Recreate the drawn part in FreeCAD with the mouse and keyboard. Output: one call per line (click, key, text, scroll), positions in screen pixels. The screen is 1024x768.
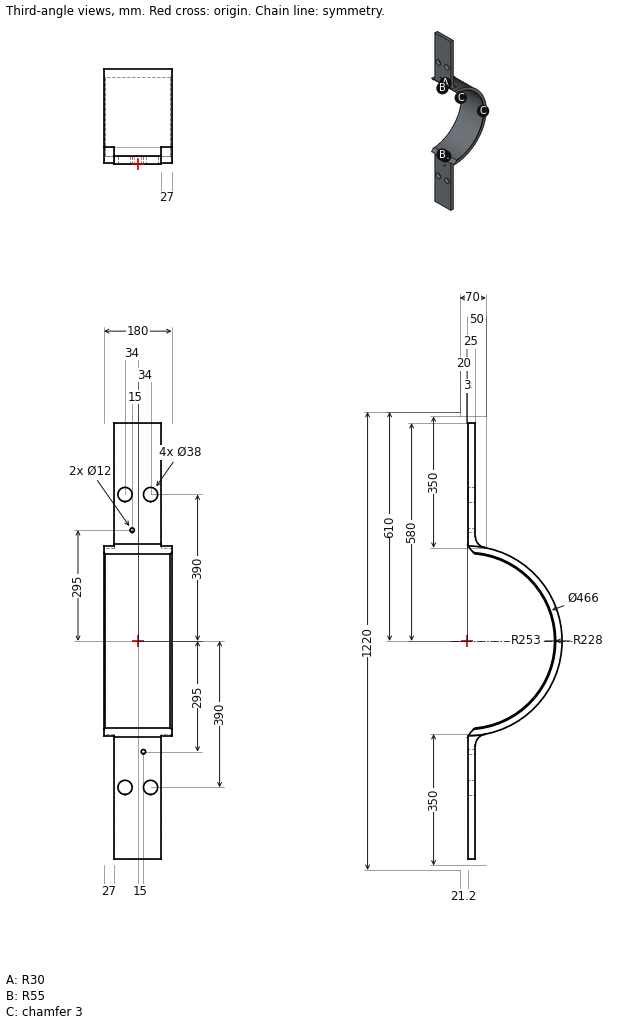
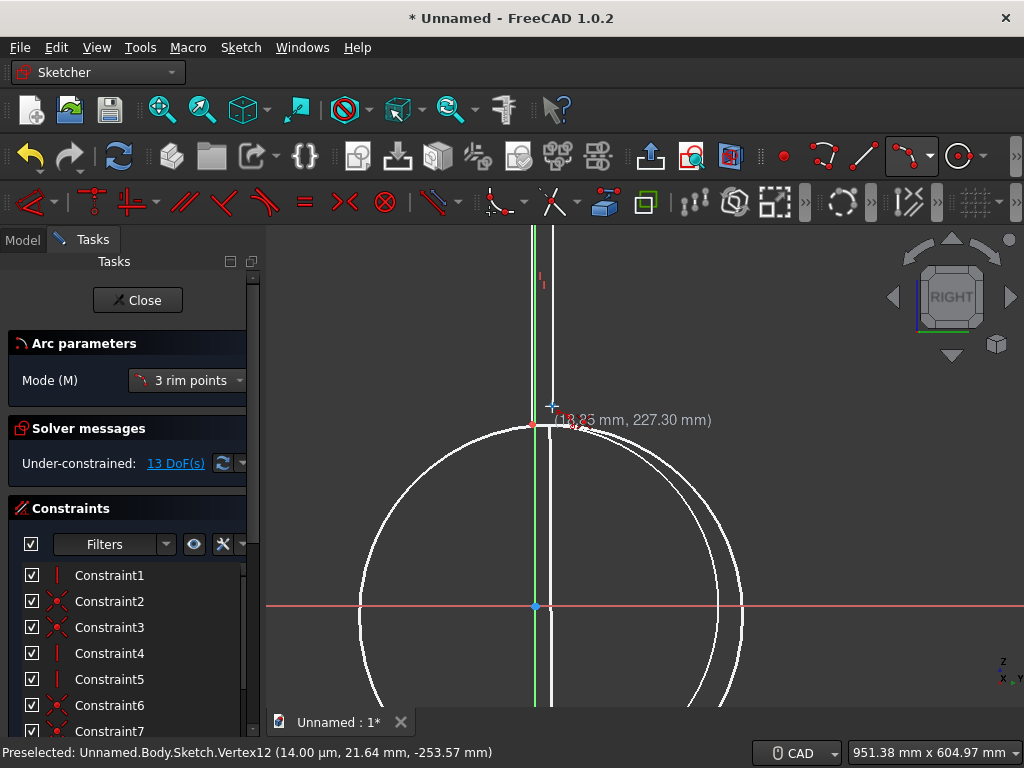
click(553, 406)
click(728, 665)
key(Escape)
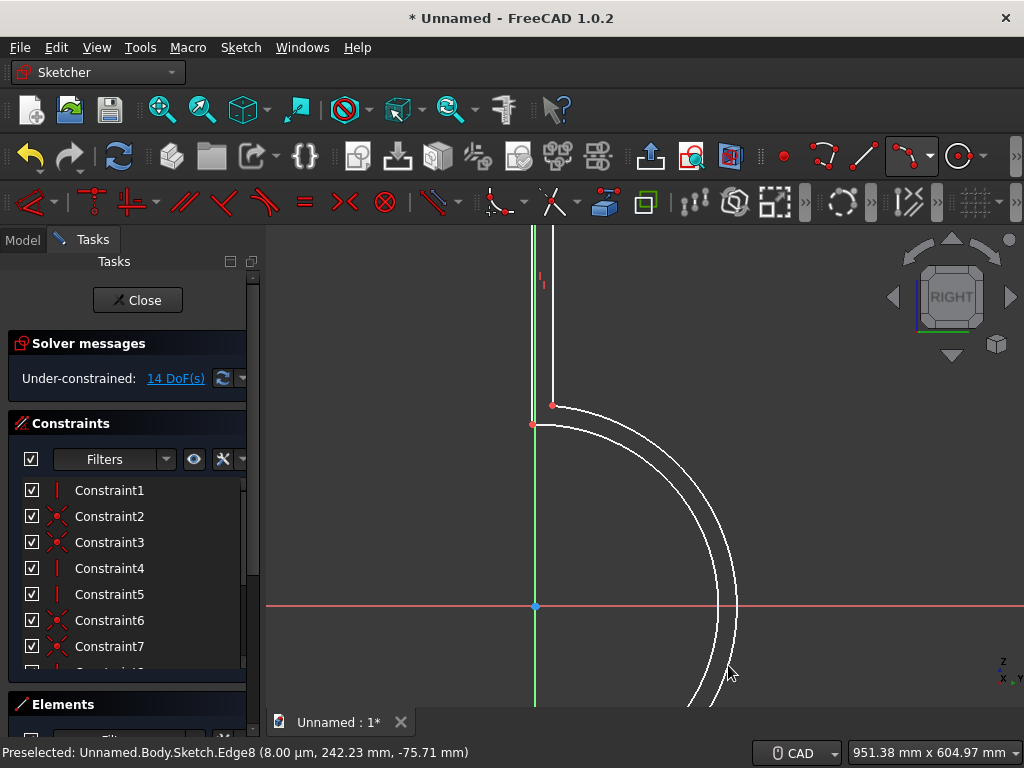
scroll(552, 406, down, 6)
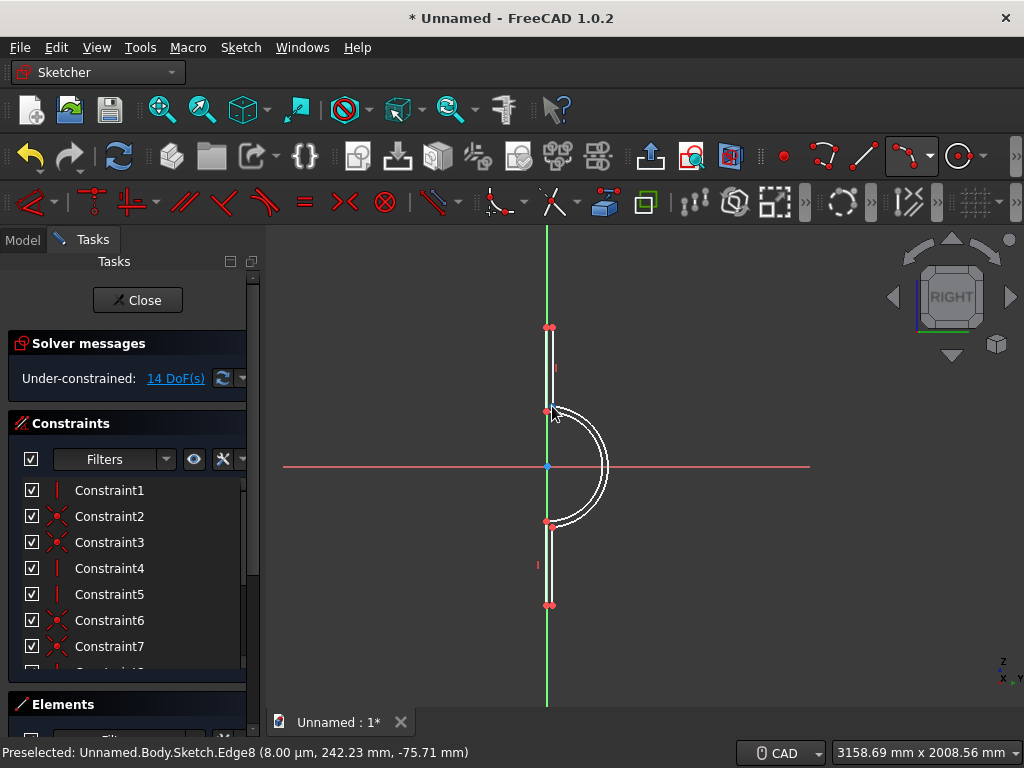
scroll(550, 328, up, 9)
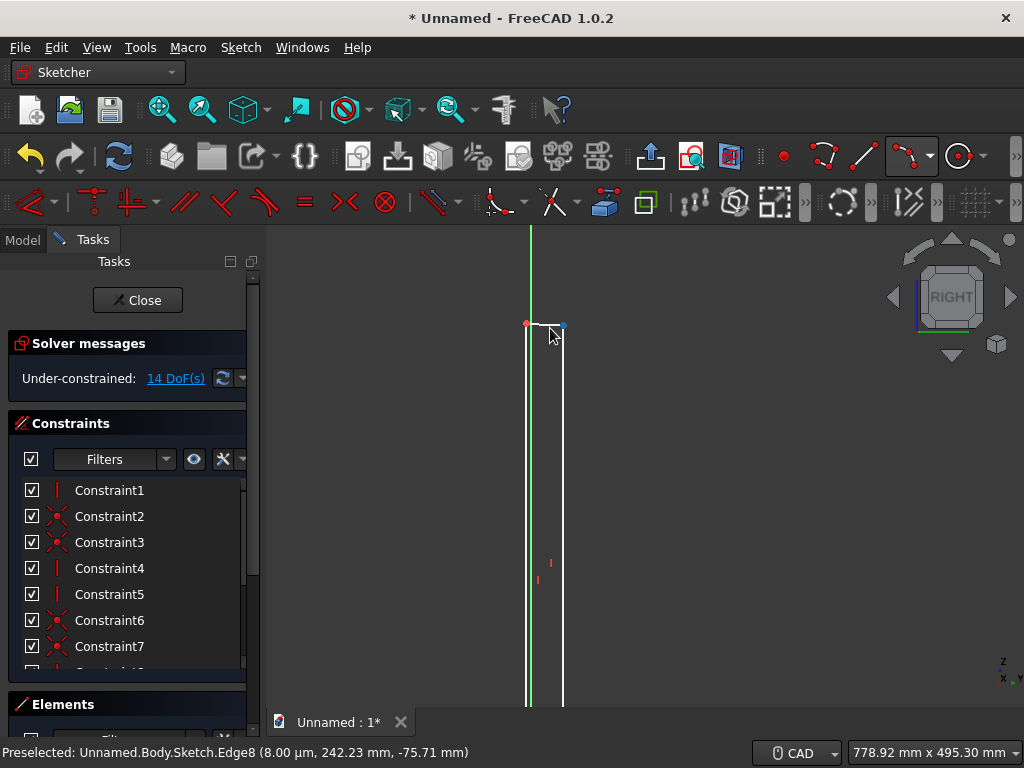
click(549, 325)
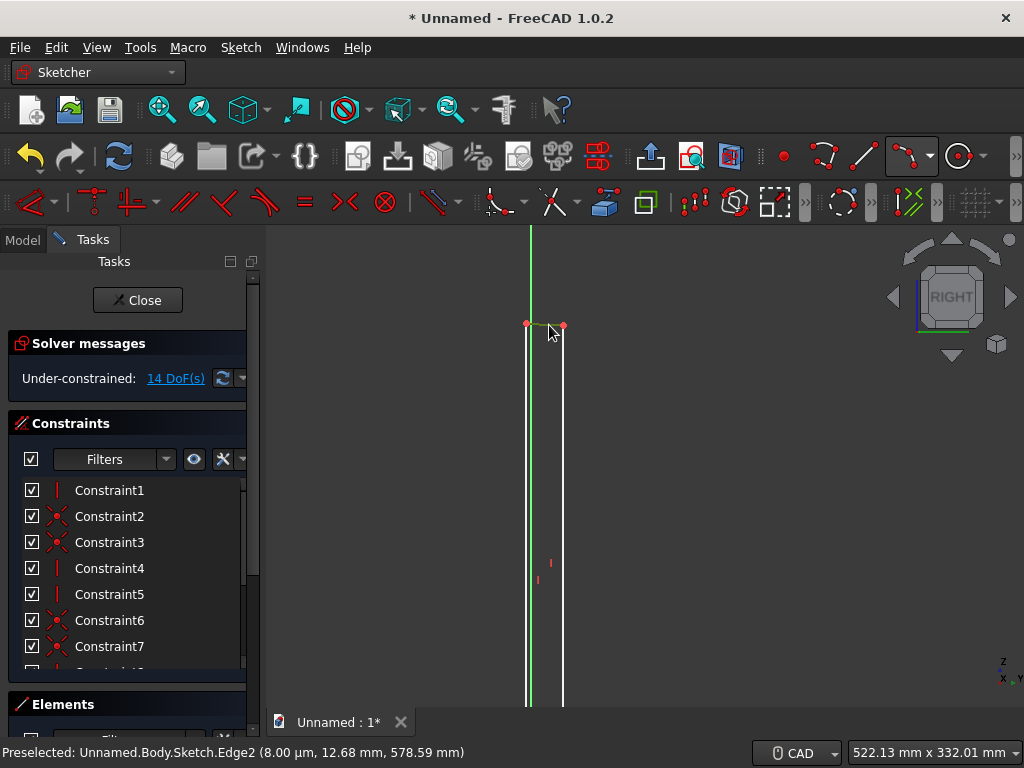
click(158, 202)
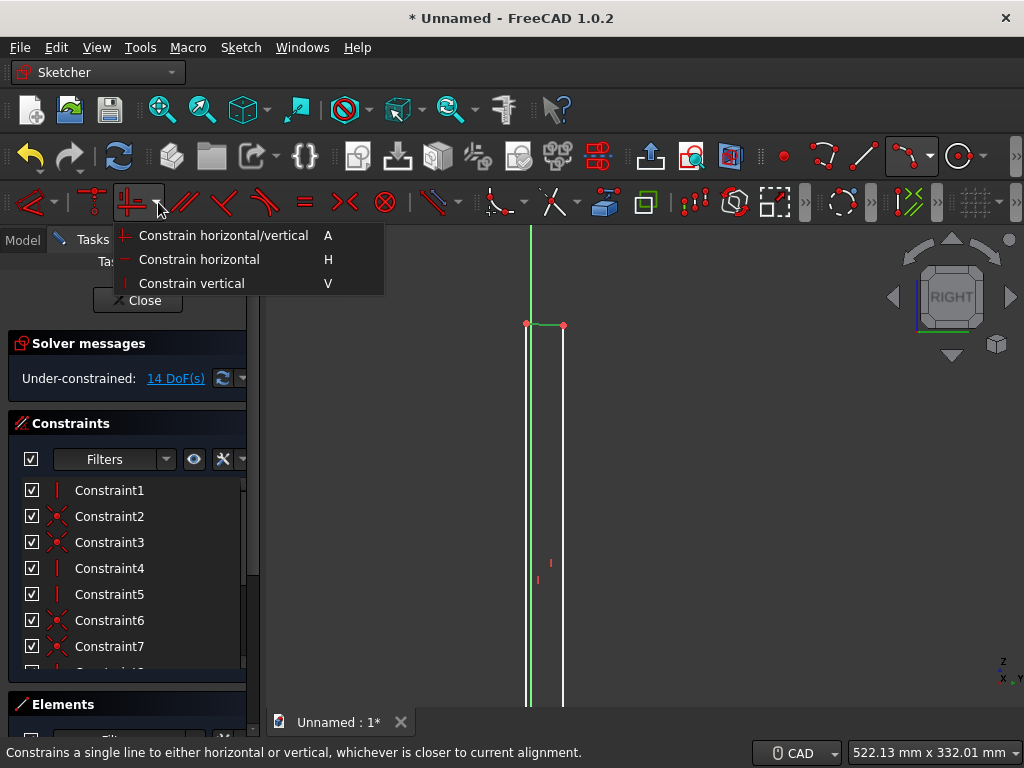
click(249, 259)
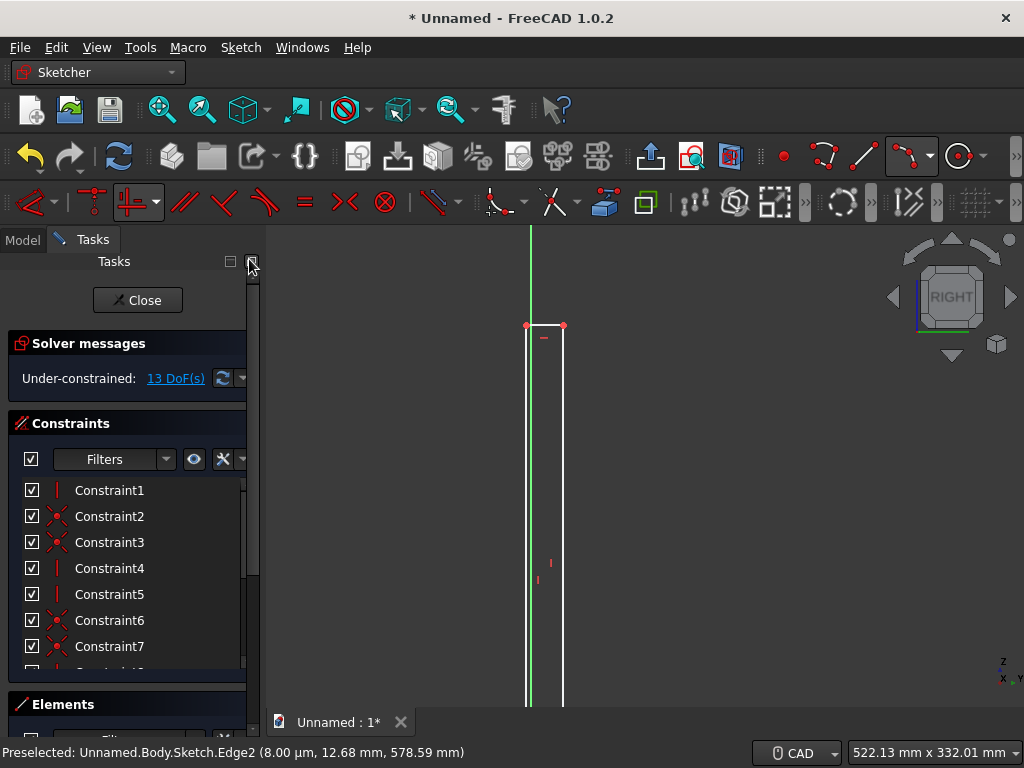
scroll(550, 328, down, 9)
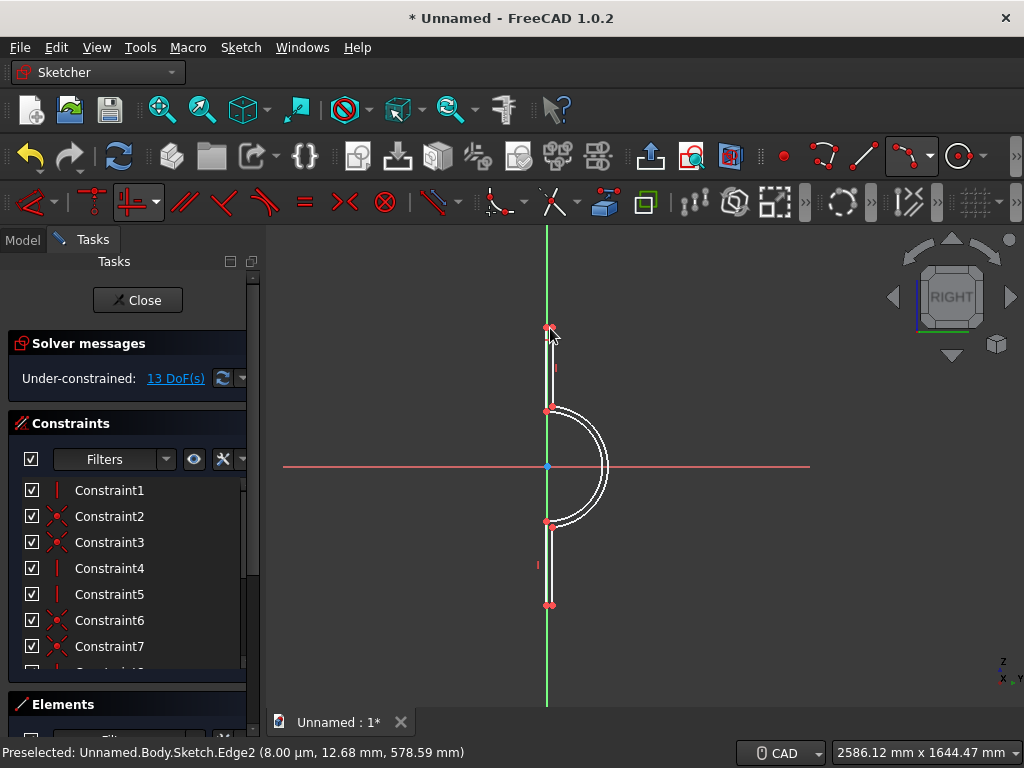
scroll(551, 606, up, 11)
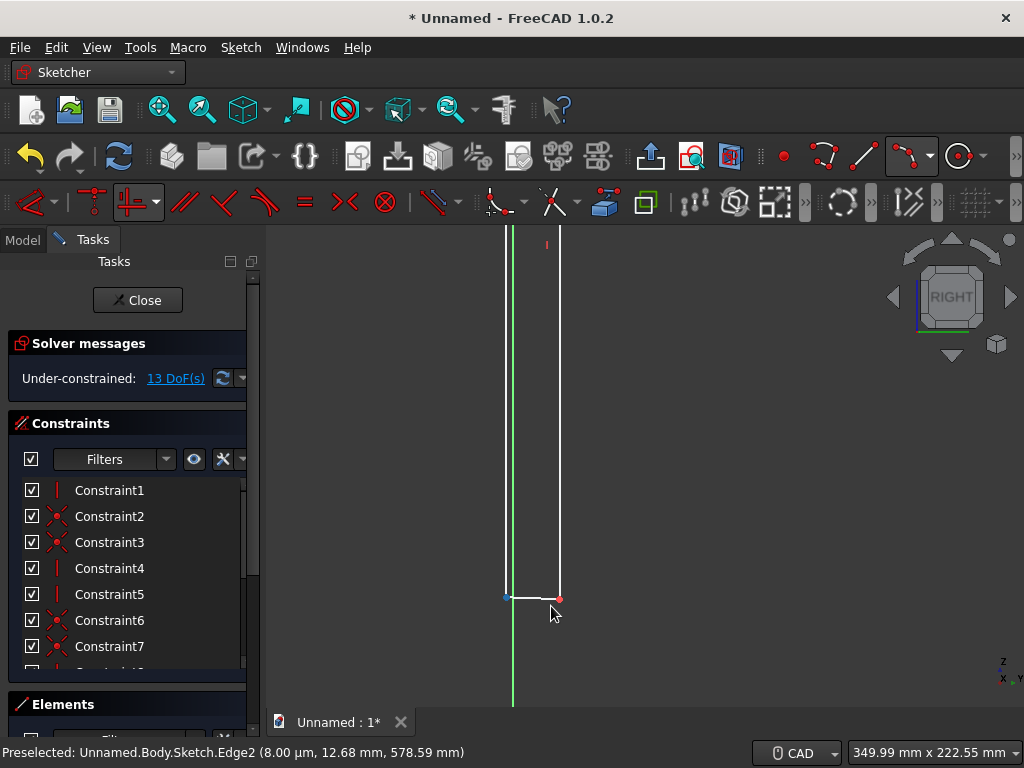
click(544, 599)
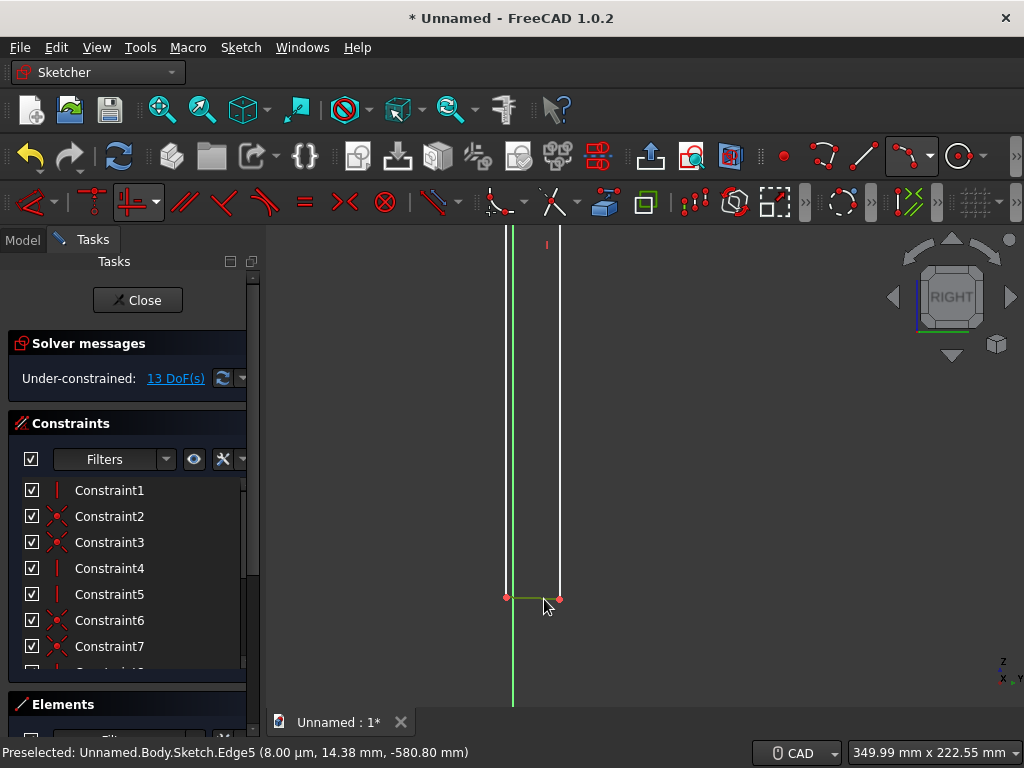
click(158, 202)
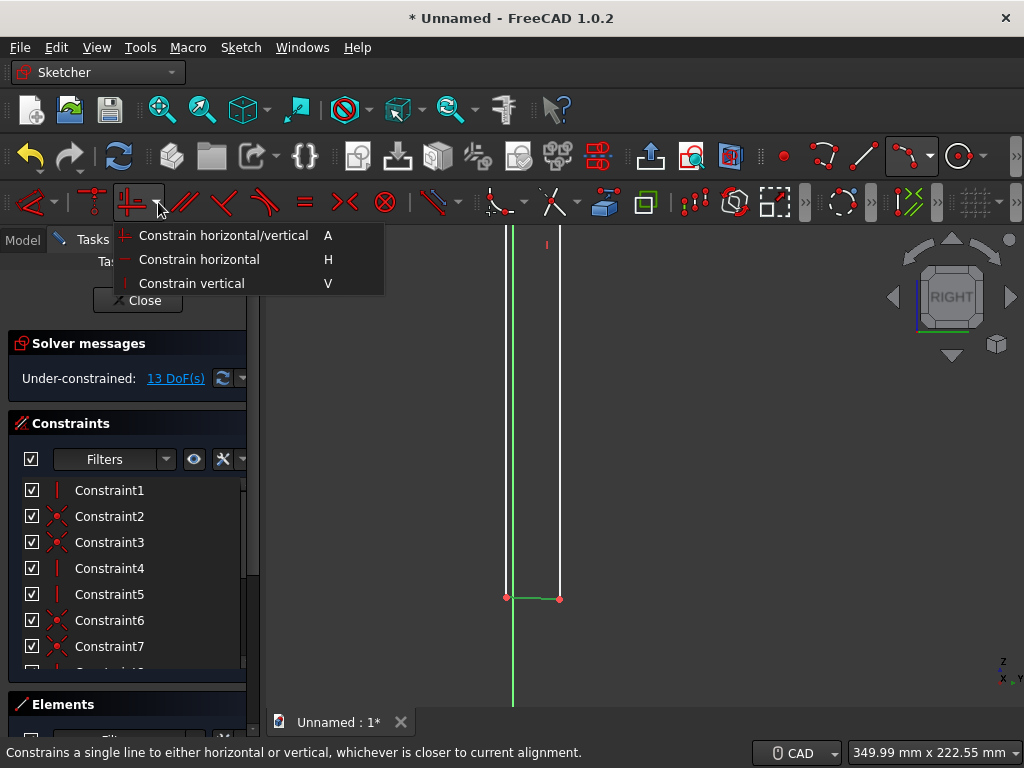
click(249, 259)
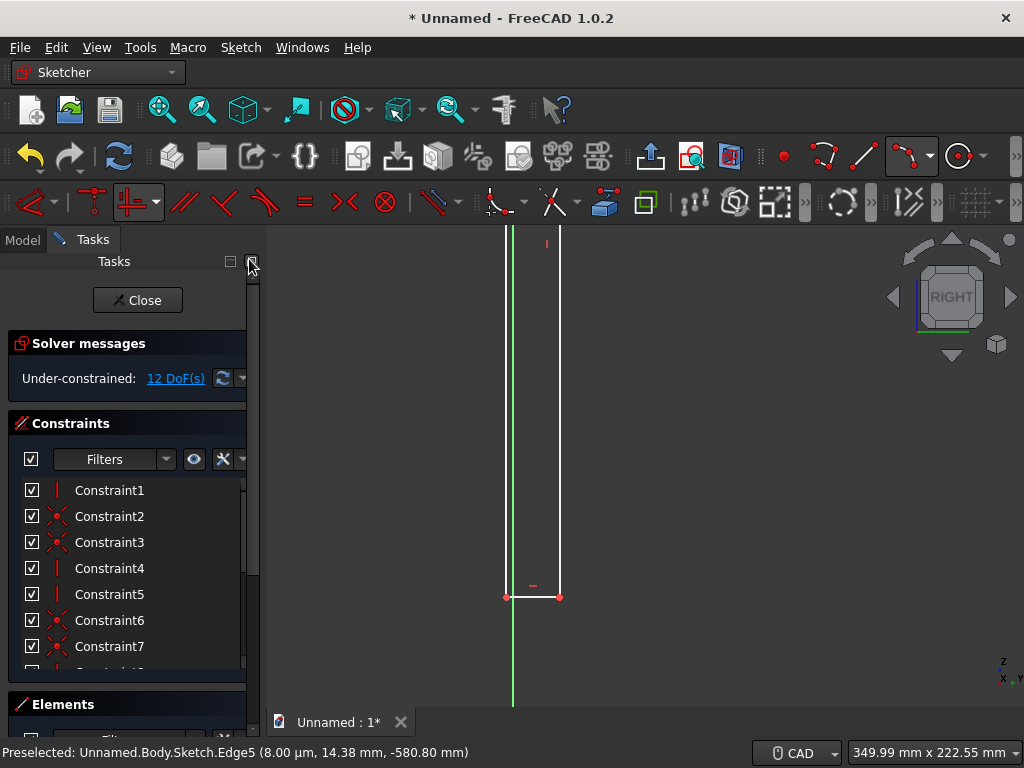
scroll(551, 606, down, 11)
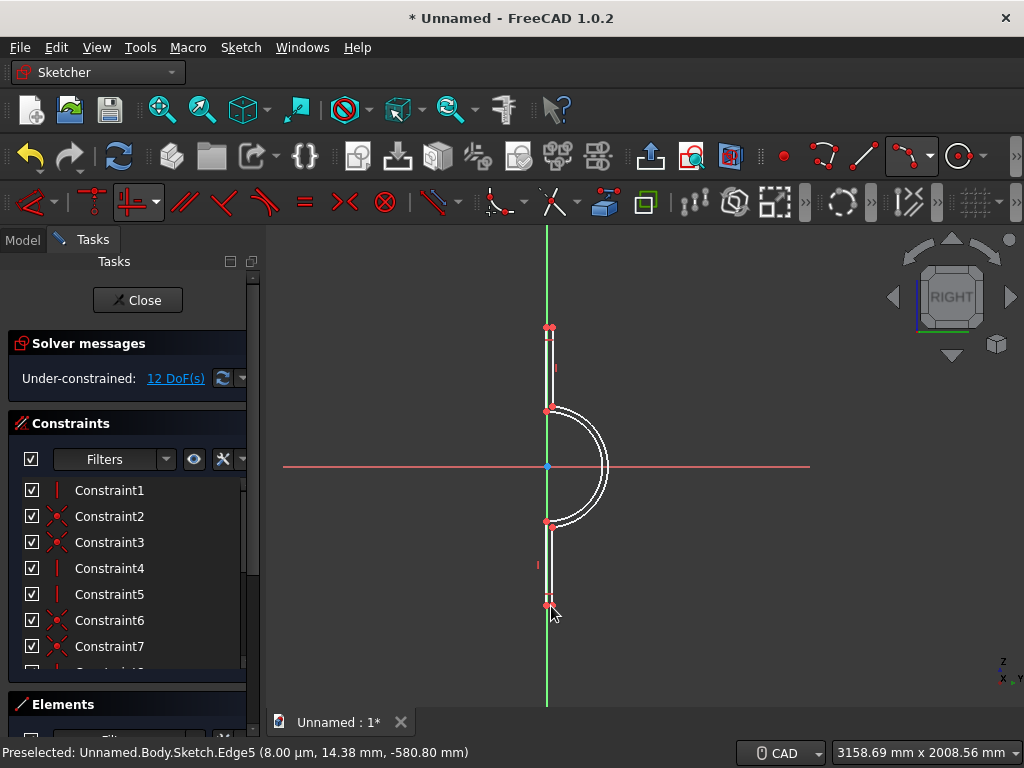
scroll(592, 499, up, 5)